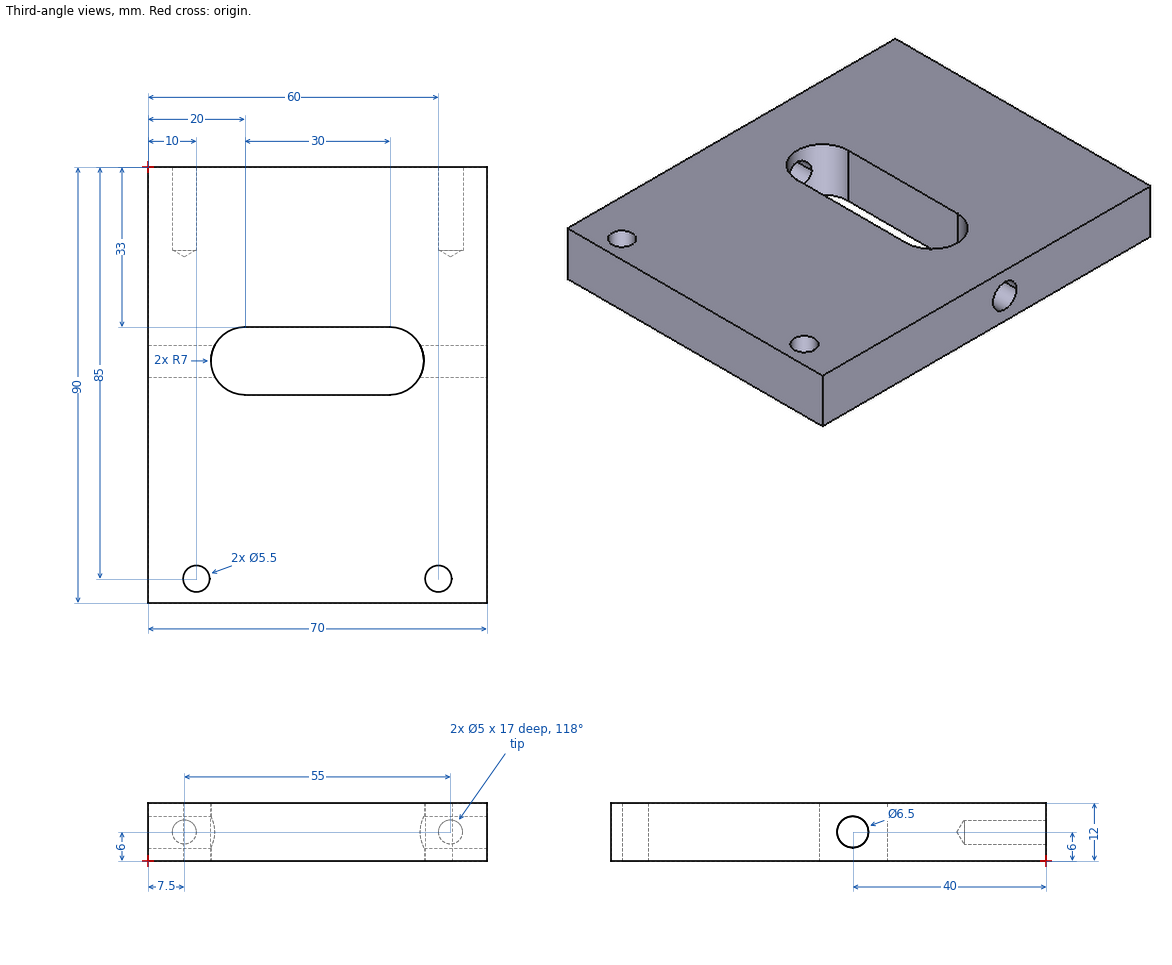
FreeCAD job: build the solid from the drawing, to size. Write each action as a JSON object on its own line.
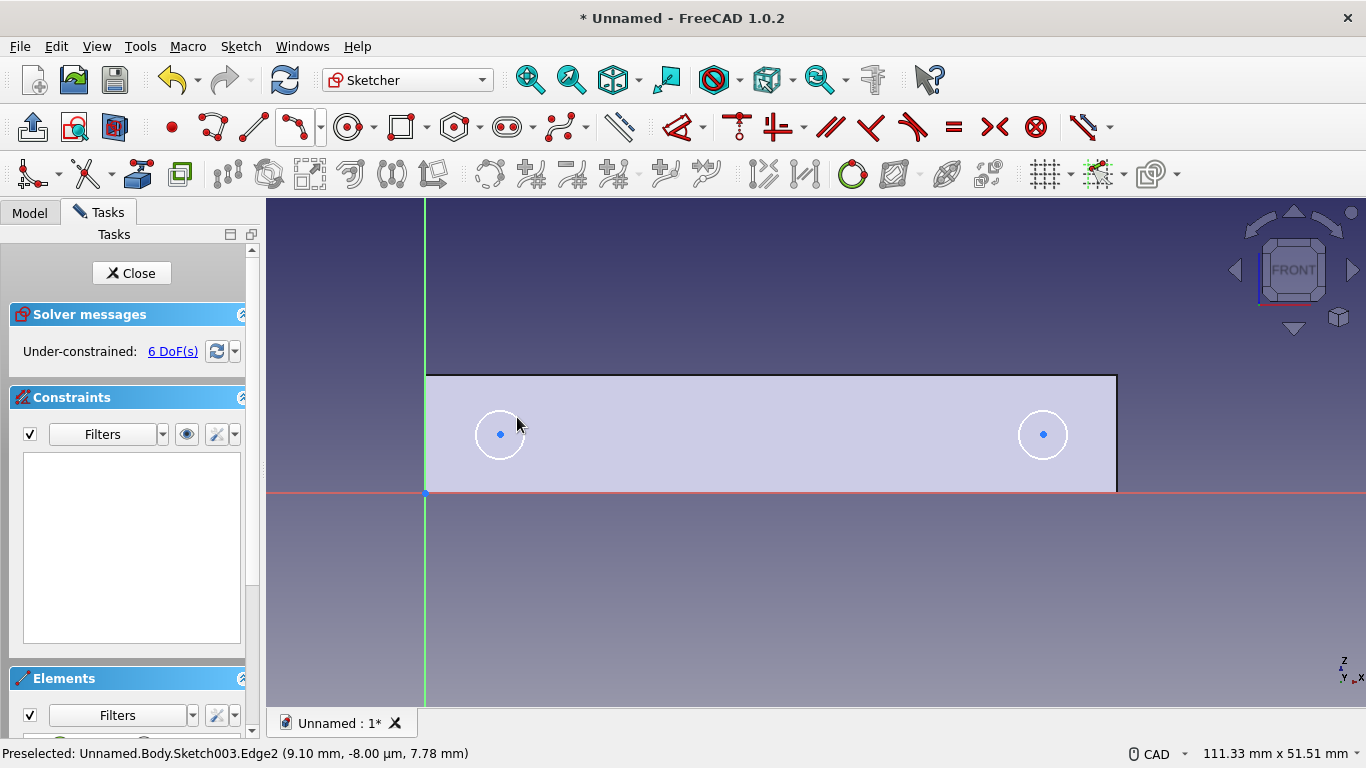
{"action": "left_click", "coordinate": [1060, 418]}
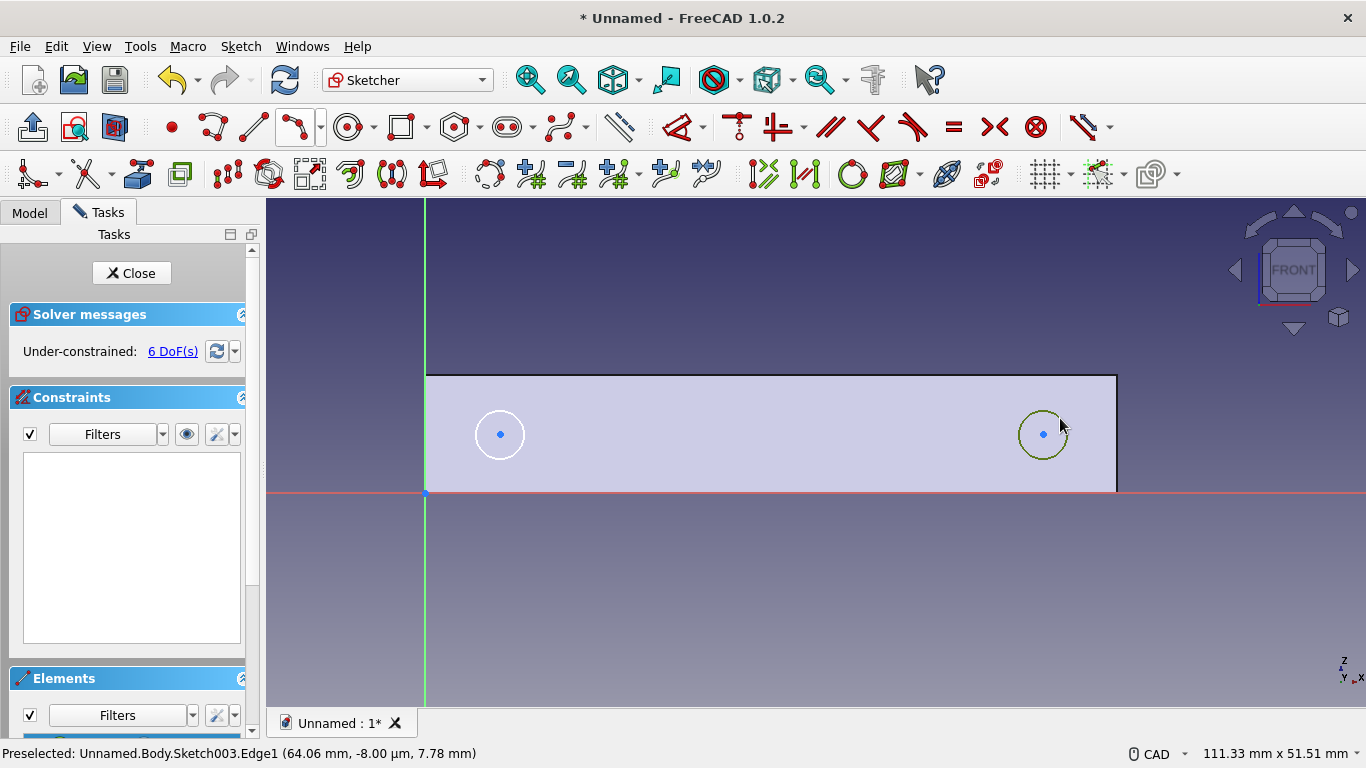
{"action": "left_click", "coordinate": [517, 418]}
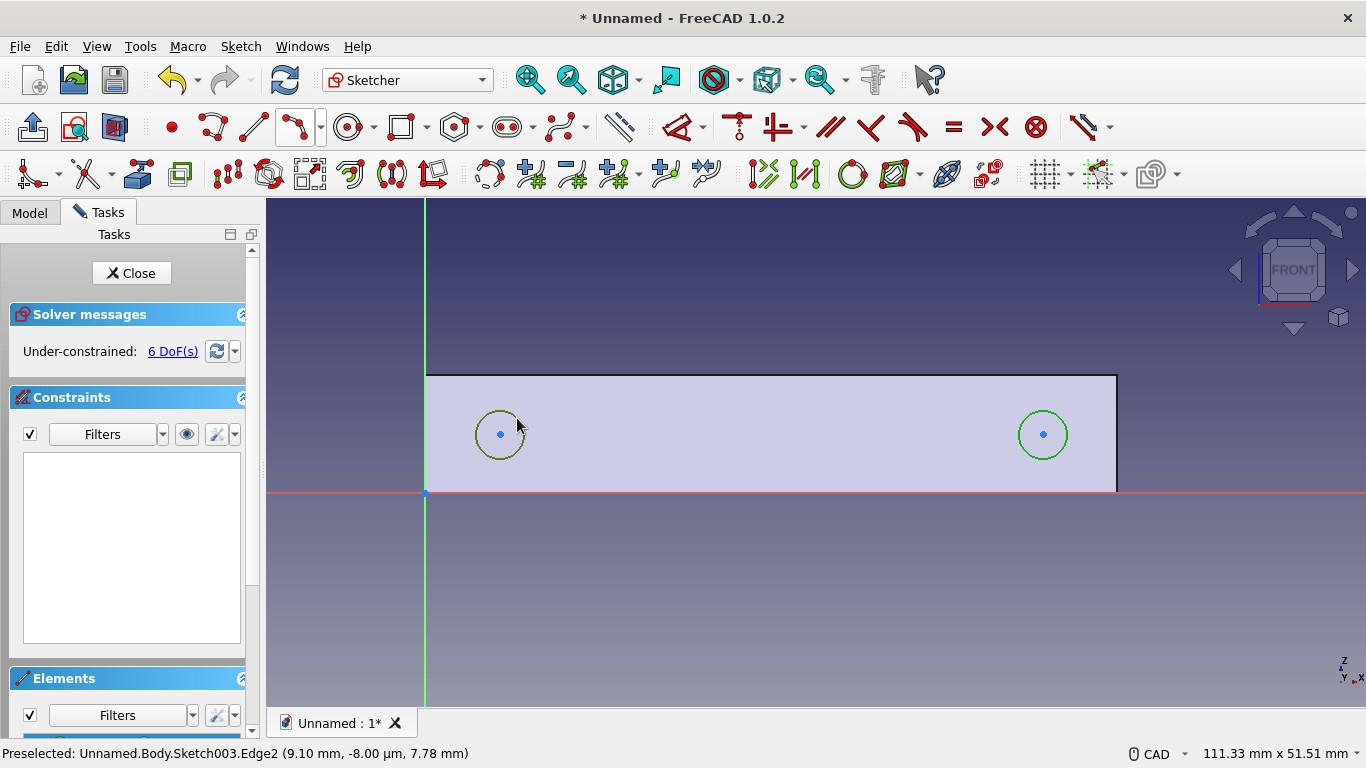
{"action": "left_click", "coordinate": [954, 128]}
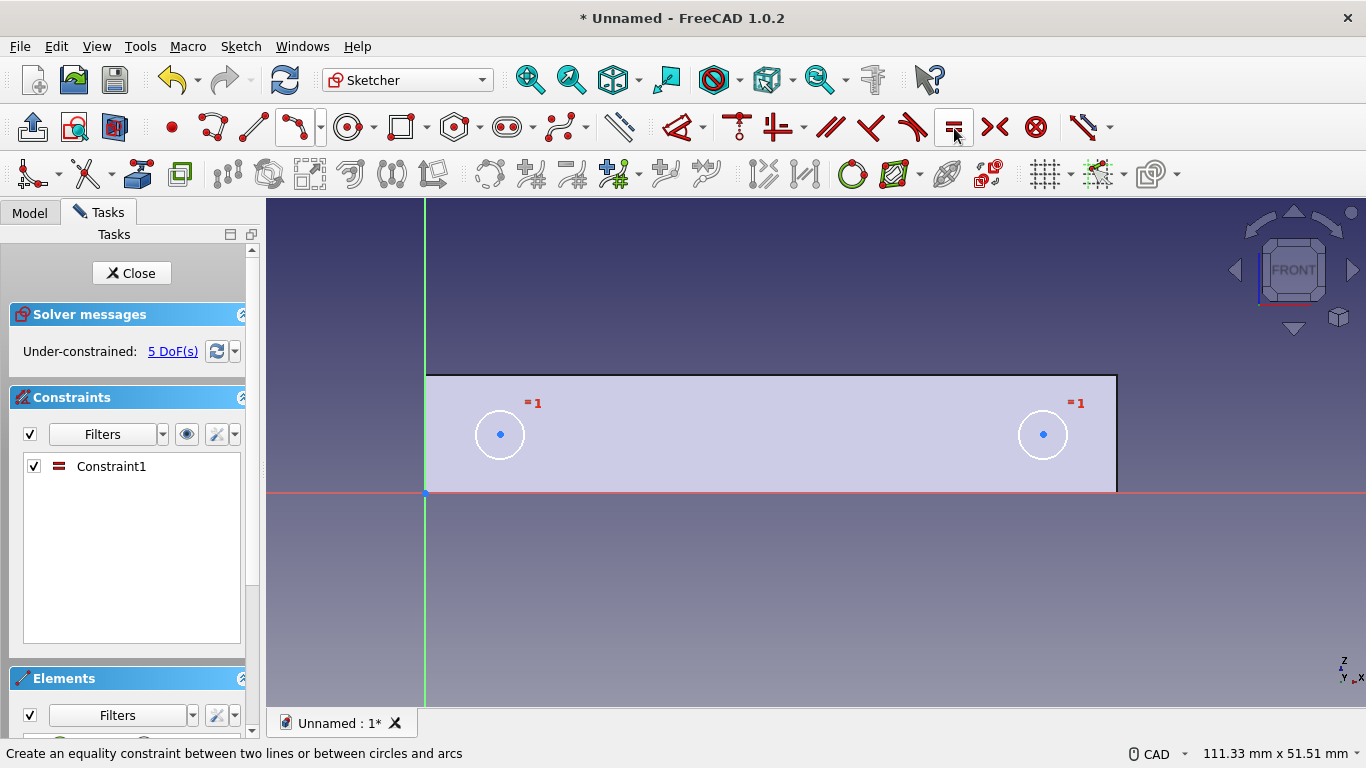
{"action": "left_click", "coordinate": [676, 128]}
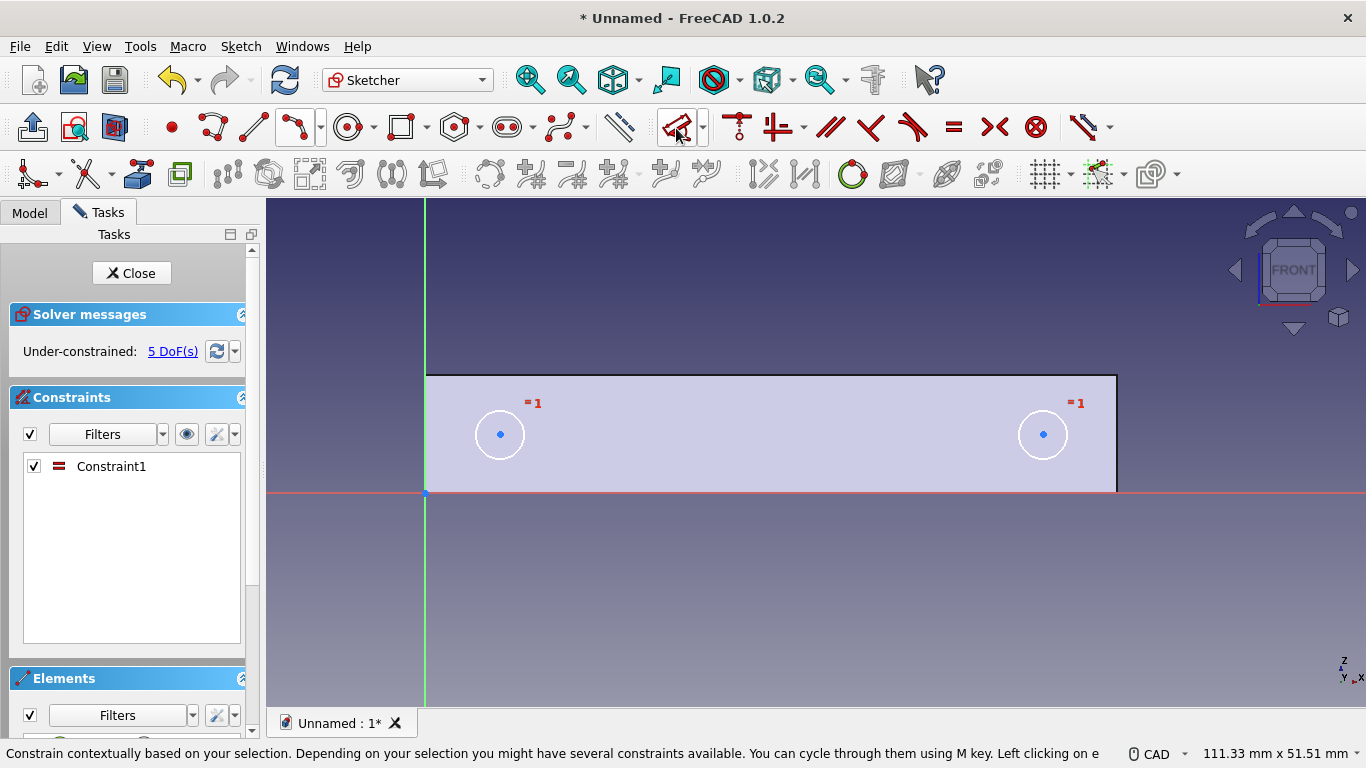
{"action": "left_click", "coordinate": [1060, 418]}
{"action": "left_click", "coordinate": [1083, 395]}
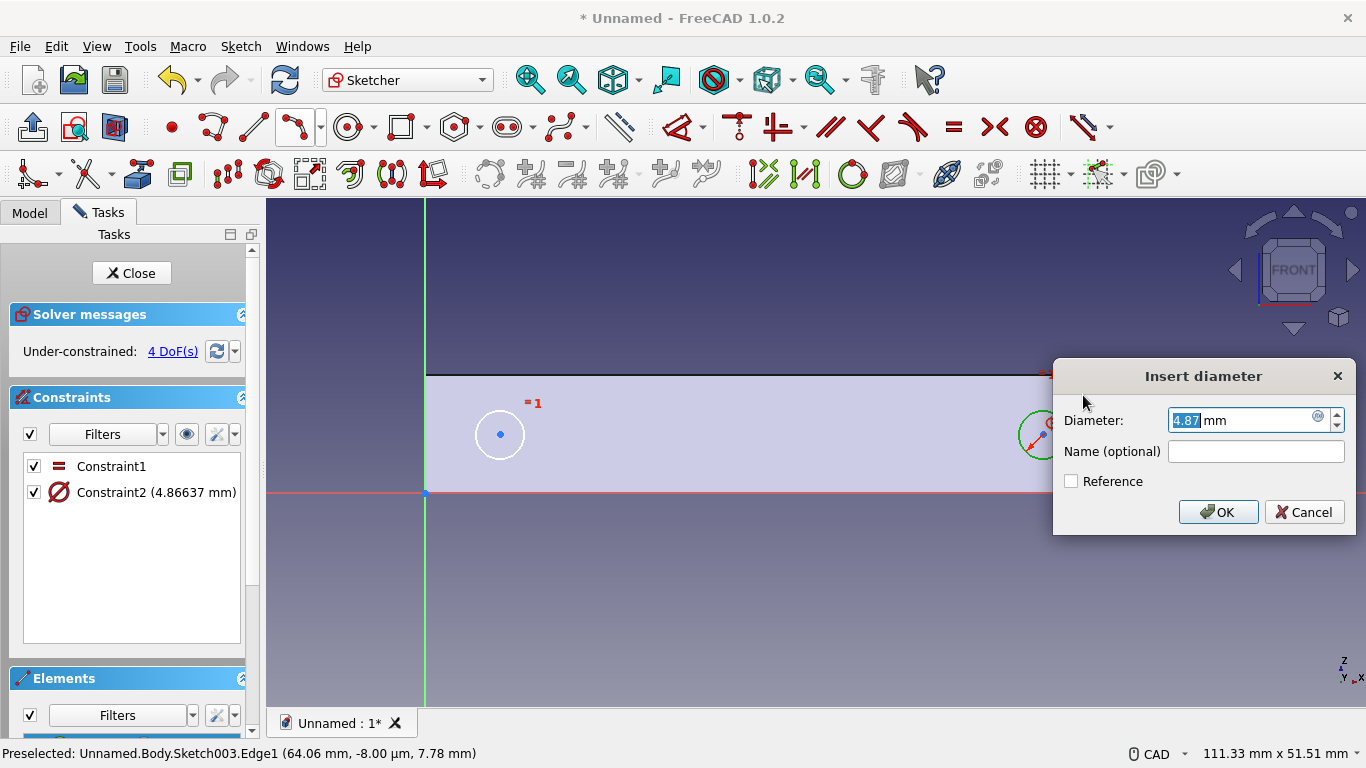
{"action": "type", "text": "5"}
{"action": "key", "text": "Return"}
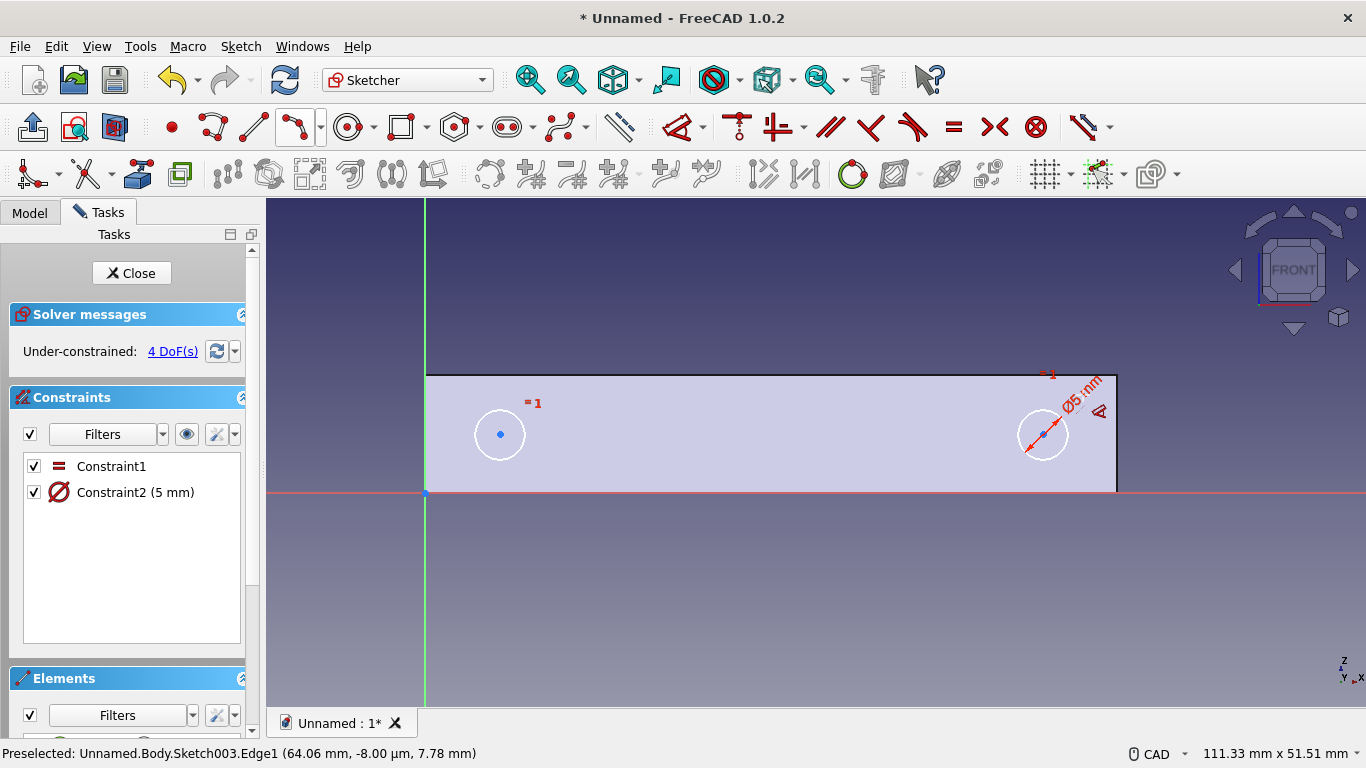
{"action": "left_click", "coordinate": [1043, 435]}
{"action": "left_click", "coordinate": [391, 464]}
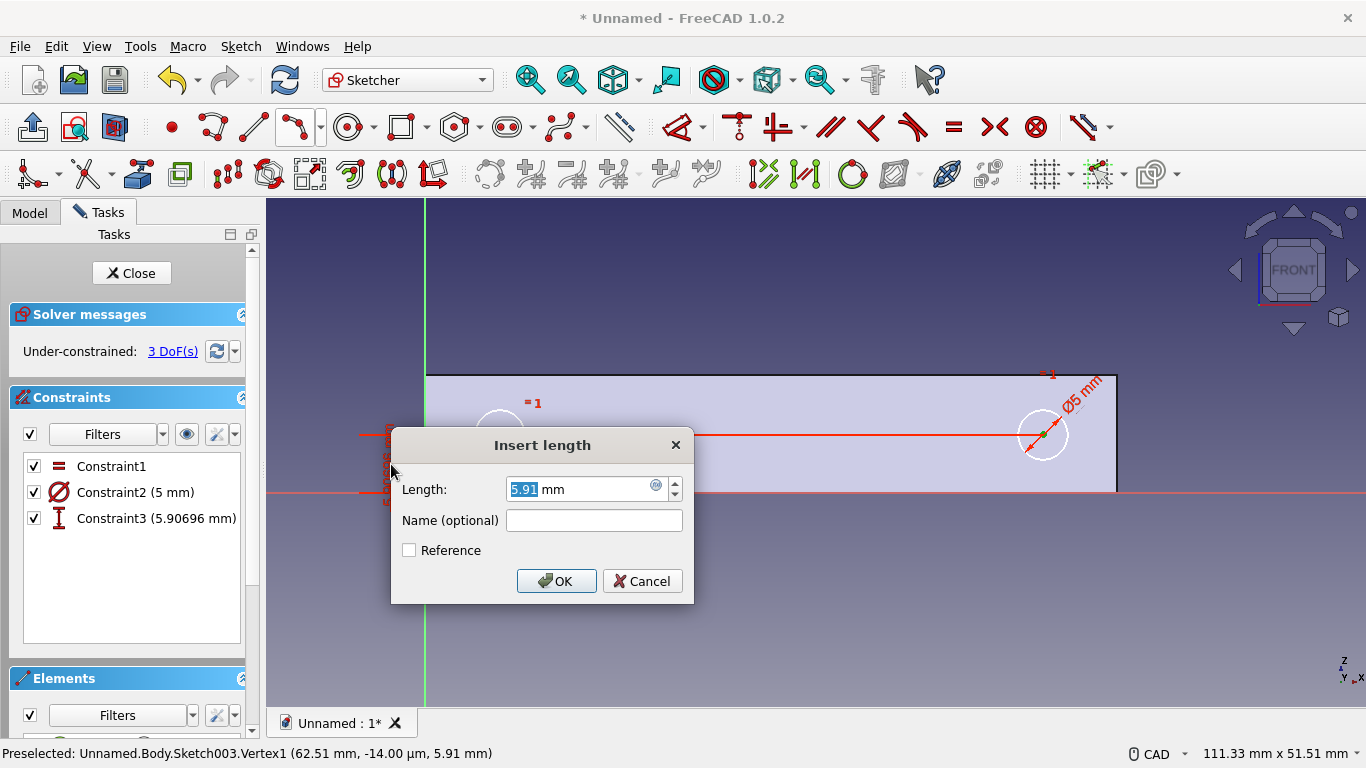
{"action": "type", "text": "6"}
{"action": "key", "text": "Return"}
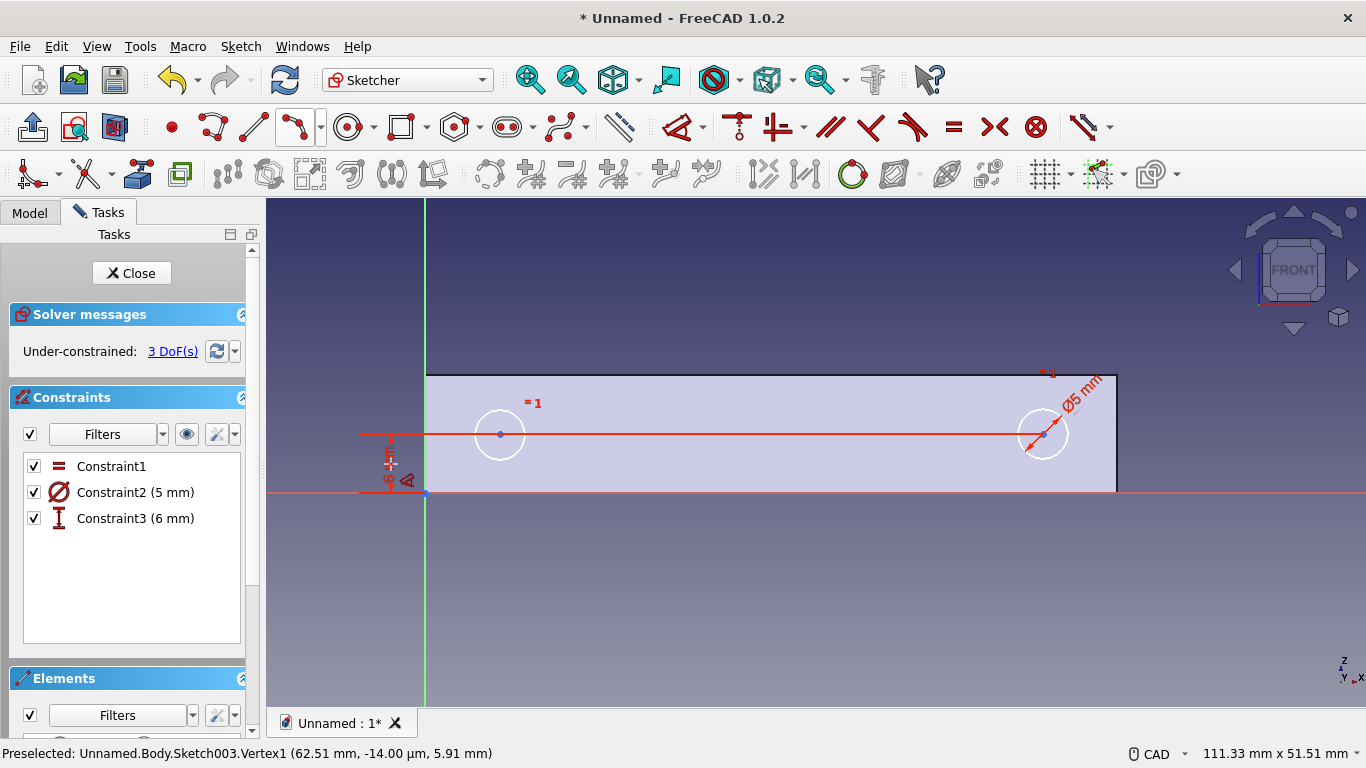
{"action": "left_click", "coordinate": [500, 435]}
{"action": "left_click", "coordinate": [391, 444]}